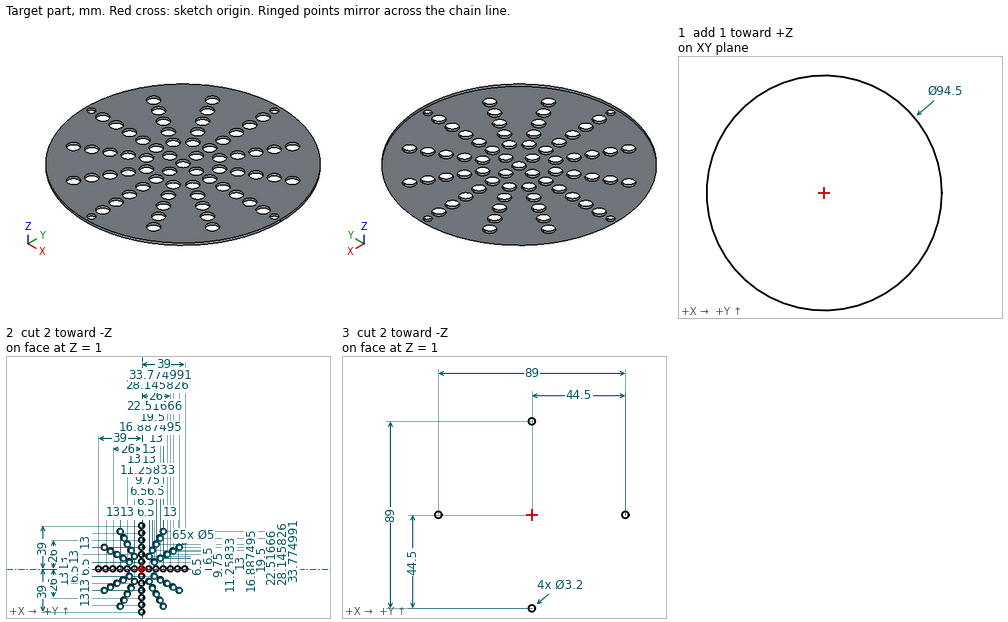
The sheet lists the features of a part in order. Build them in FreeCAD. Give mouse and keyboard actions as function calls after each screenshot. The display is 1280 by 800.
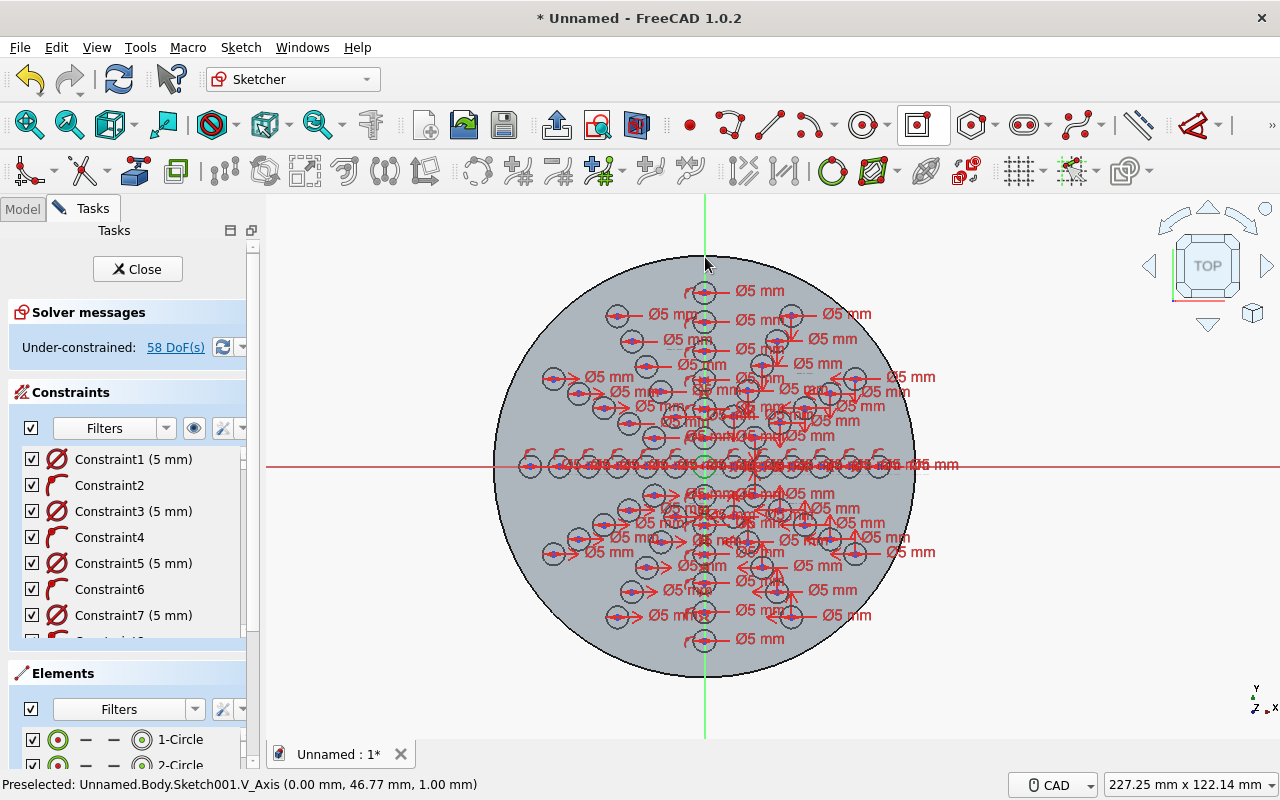
click(780, 423)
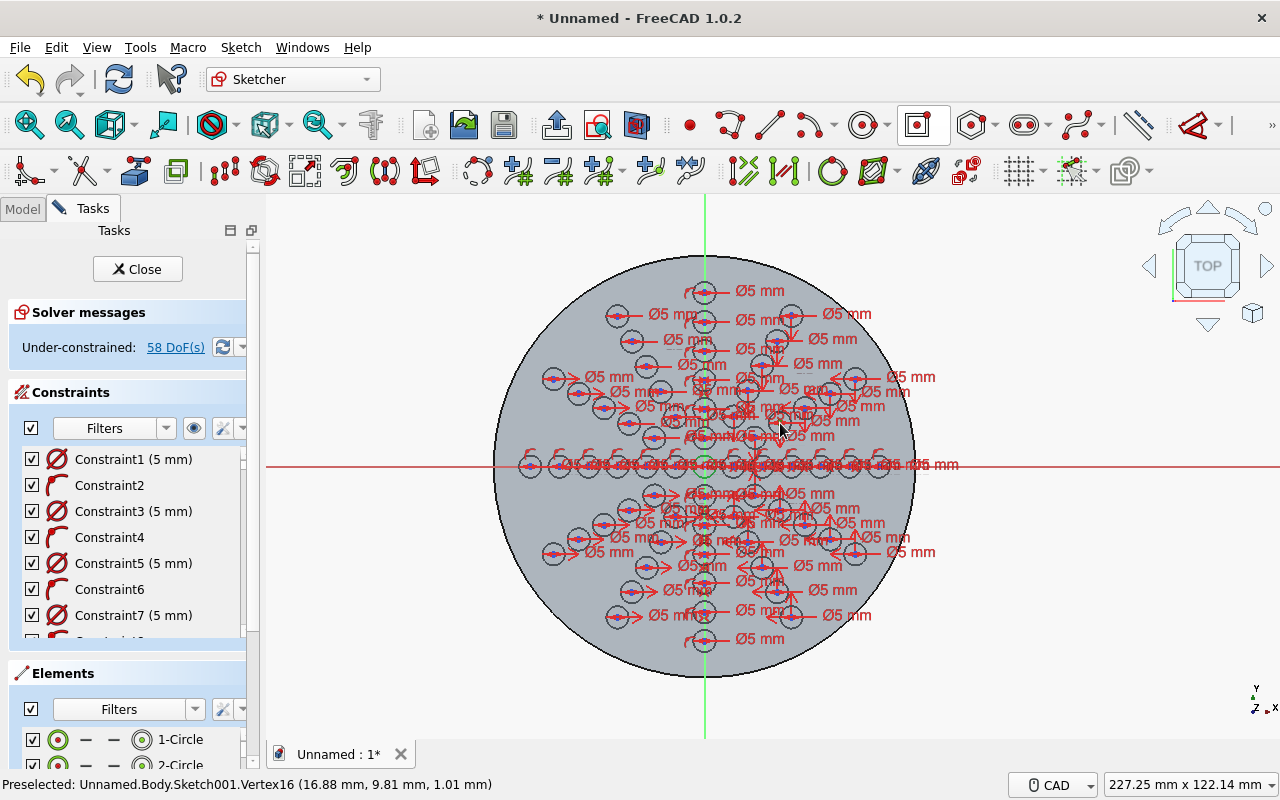
click(629, 424)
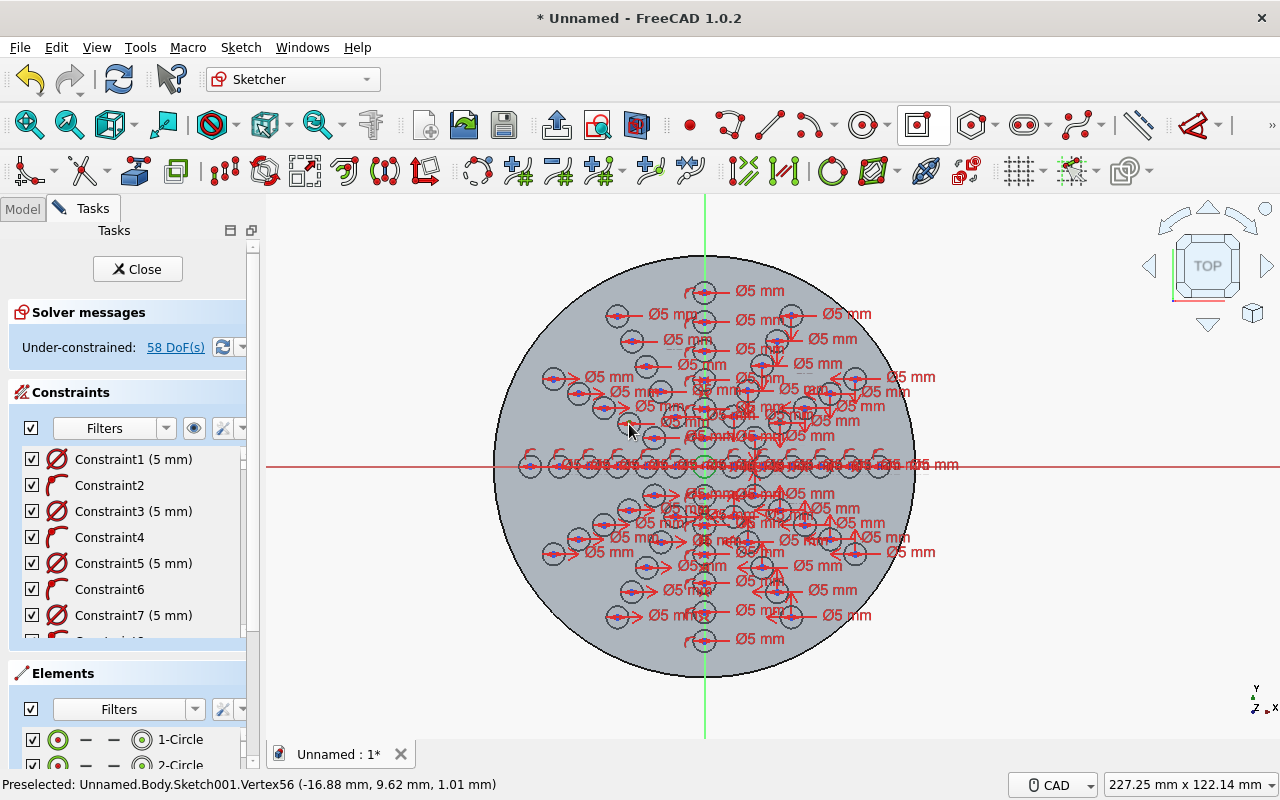
click(705, 257)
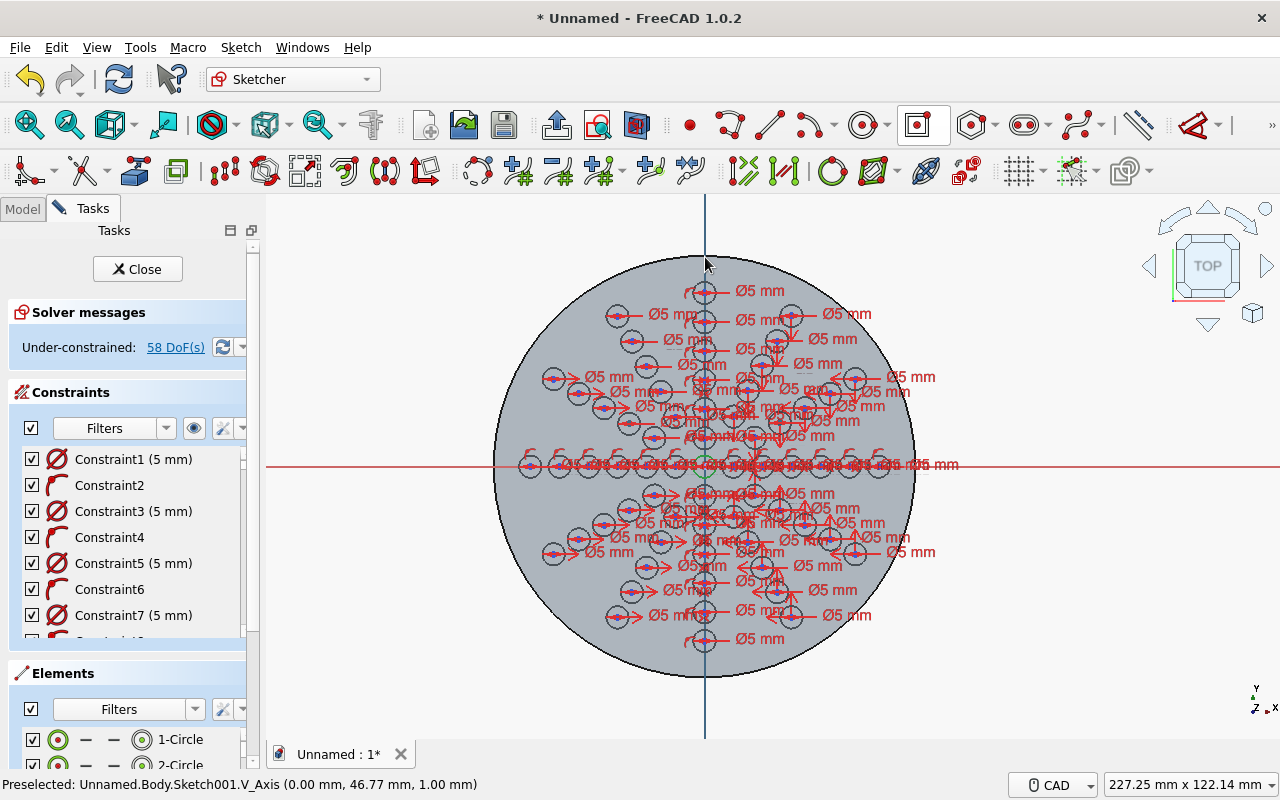
key(s)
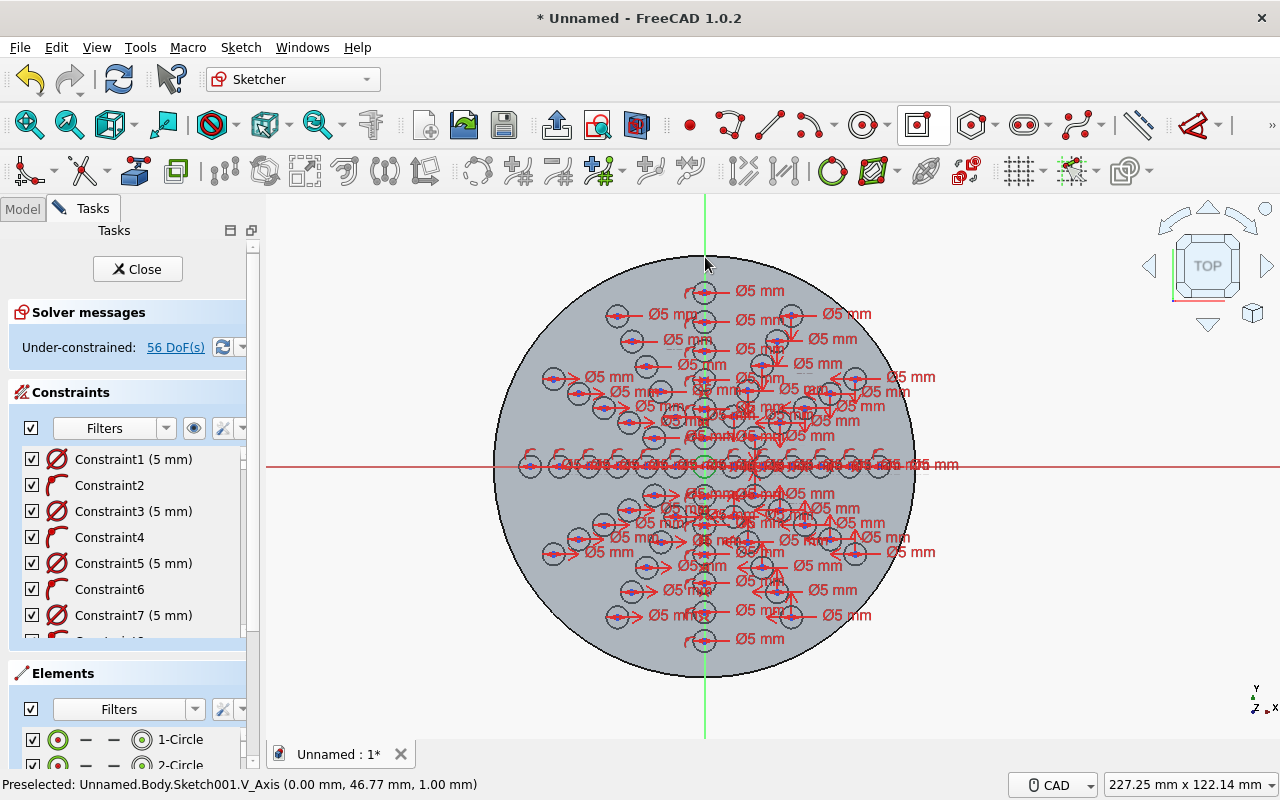
click(755, 438)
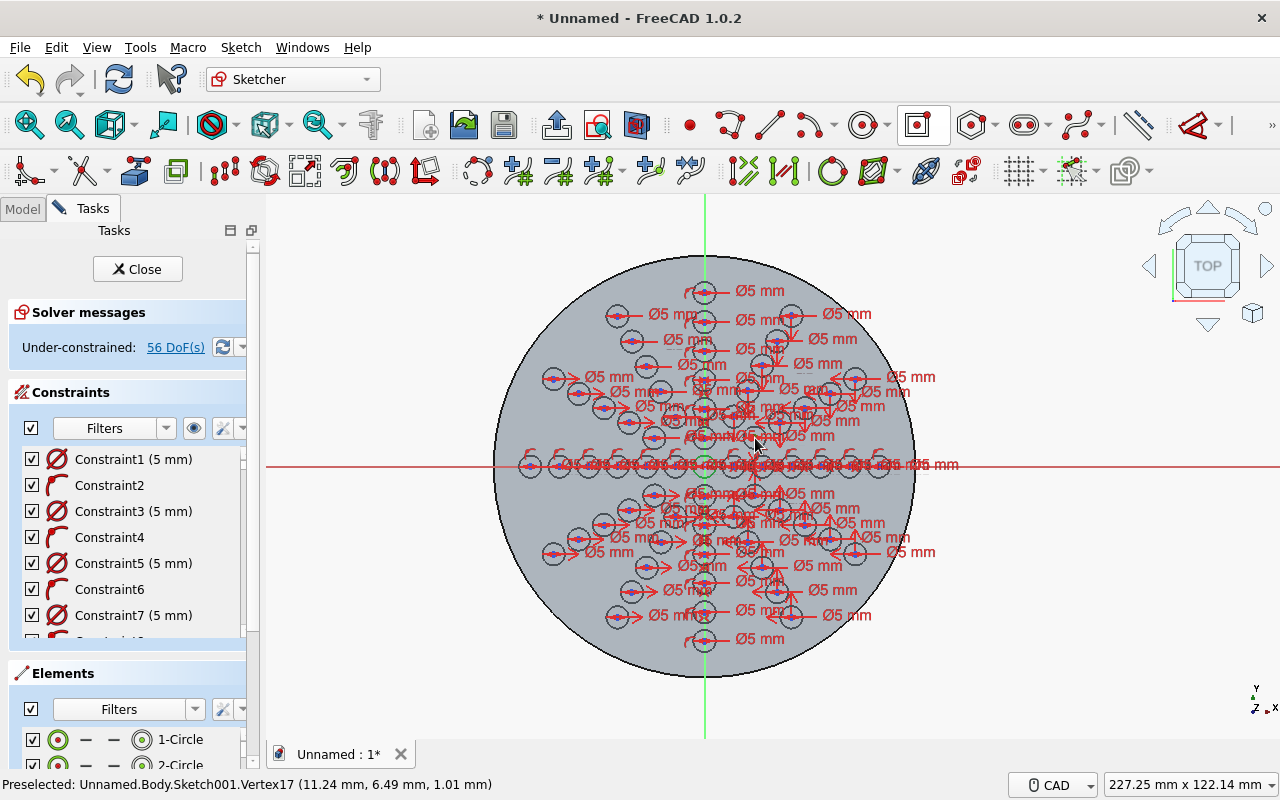
click(654, 438)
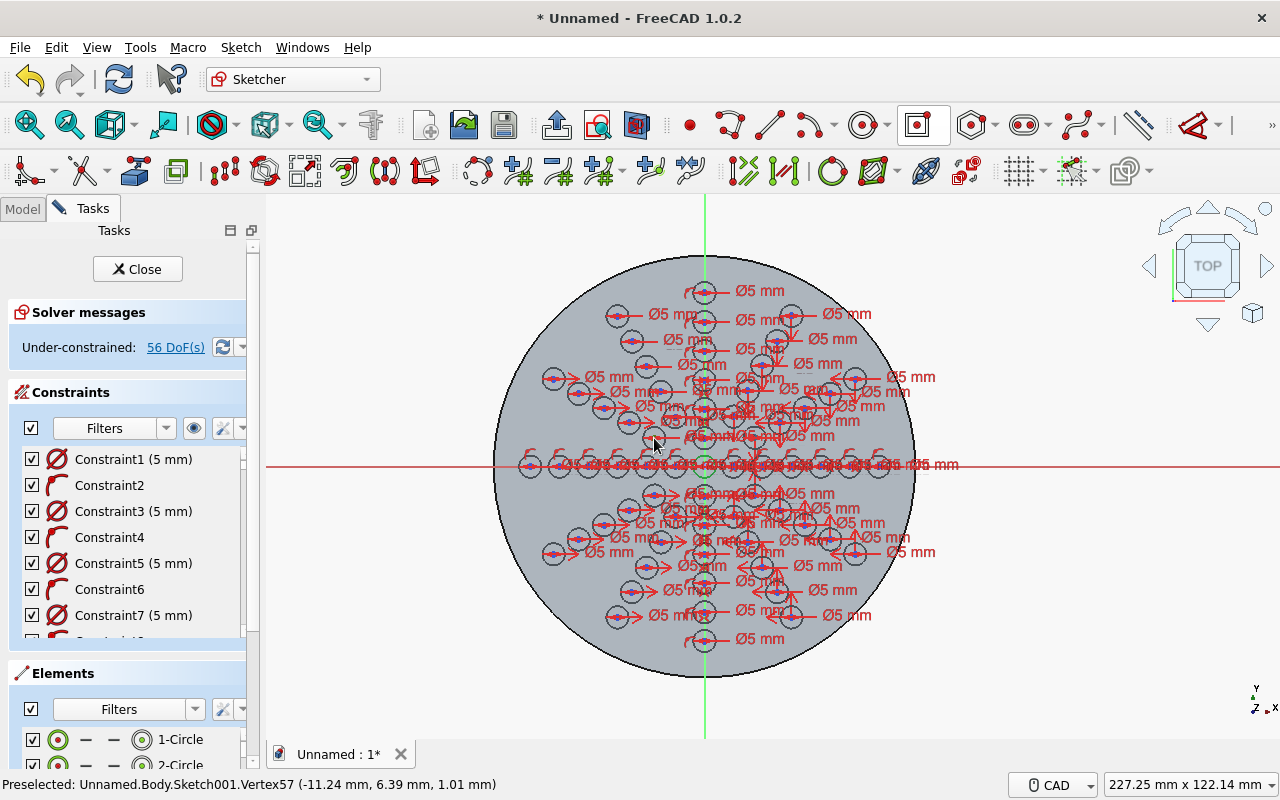
click(705, 257)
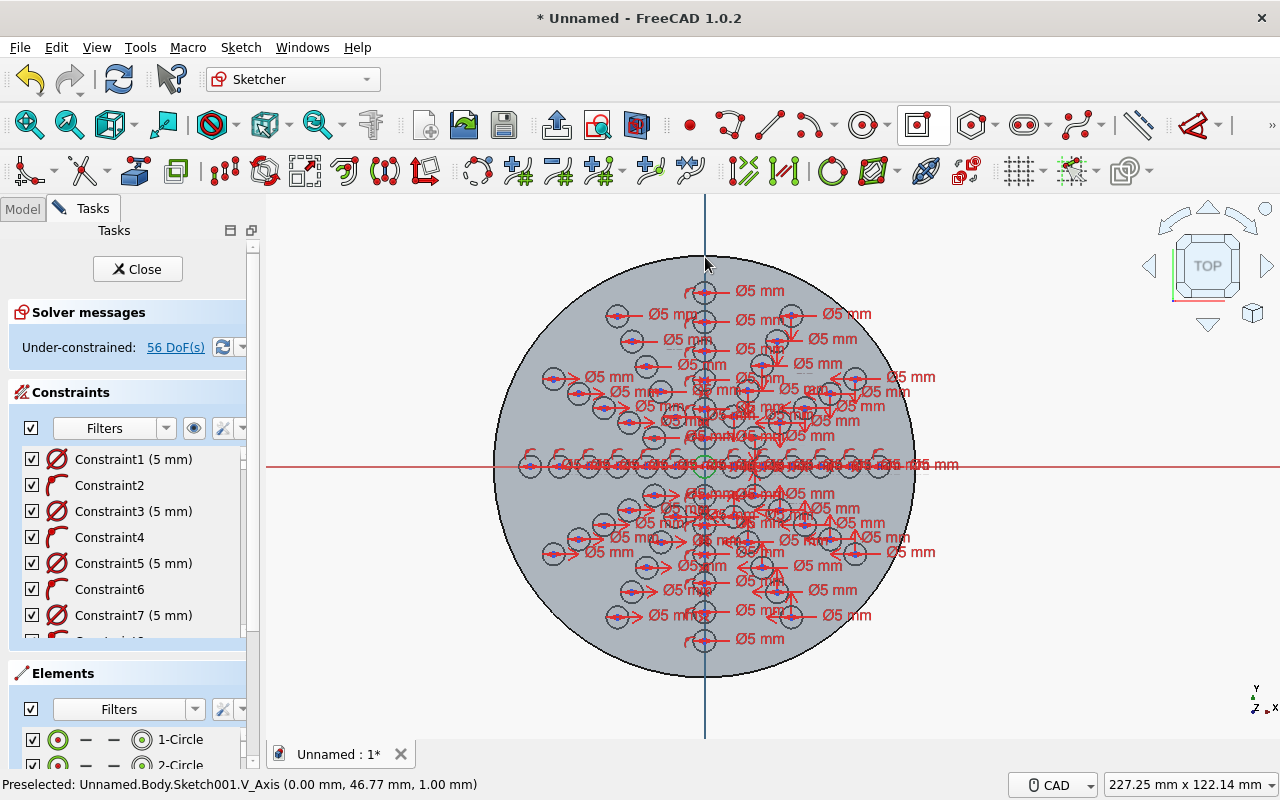
key(s)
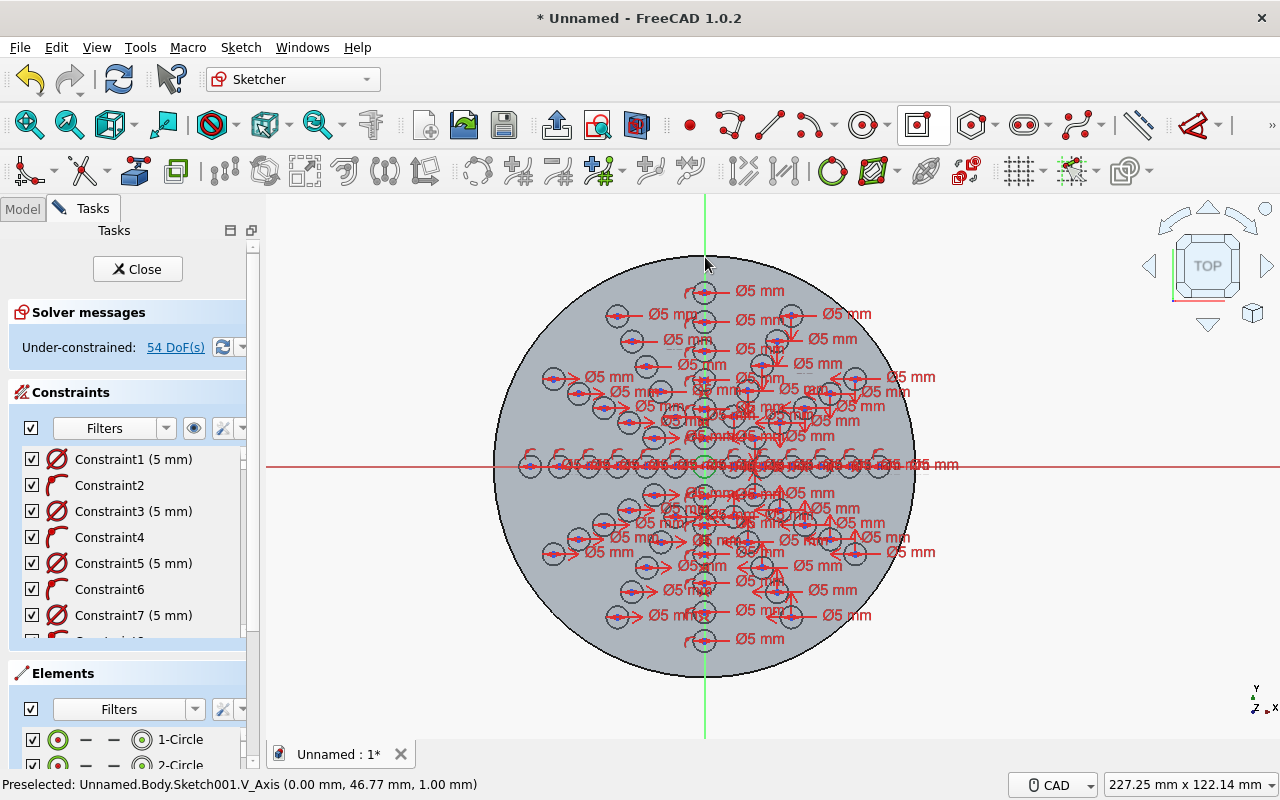
click(791, 316)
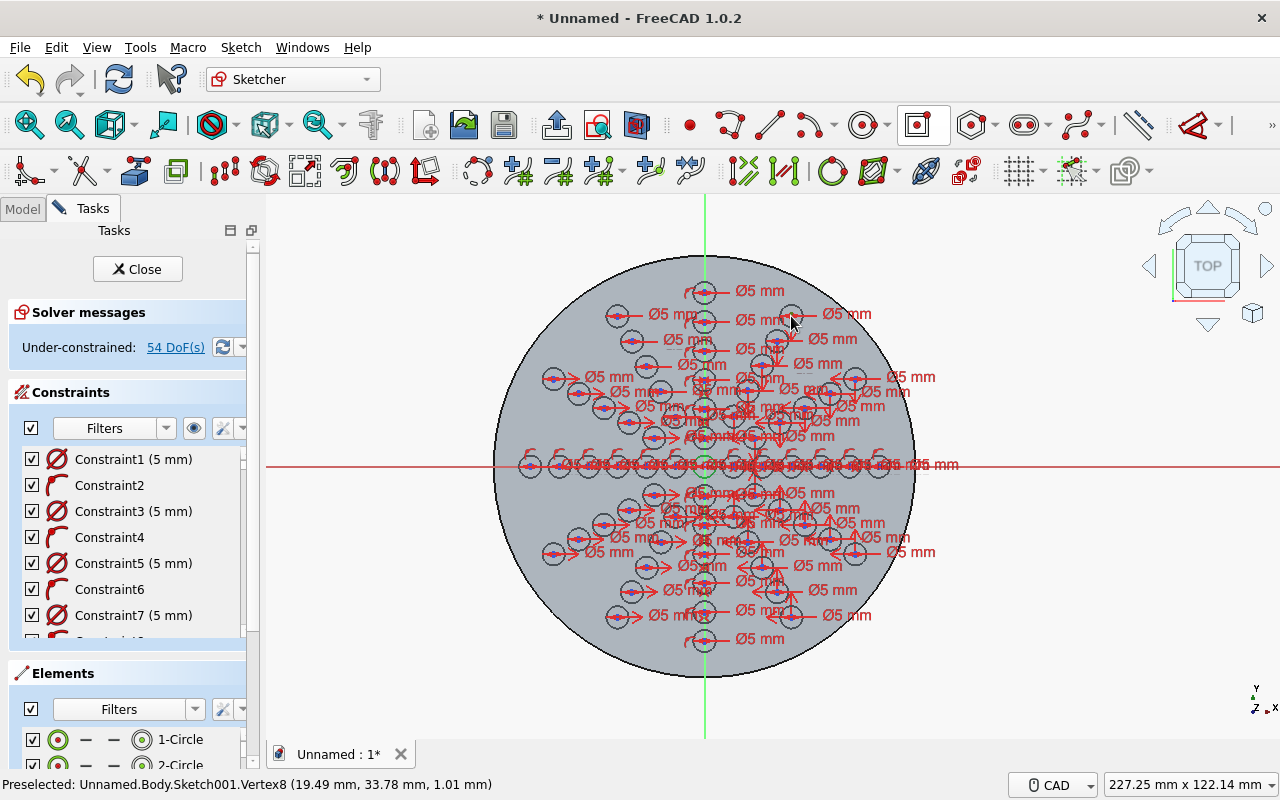
click(618, 316)